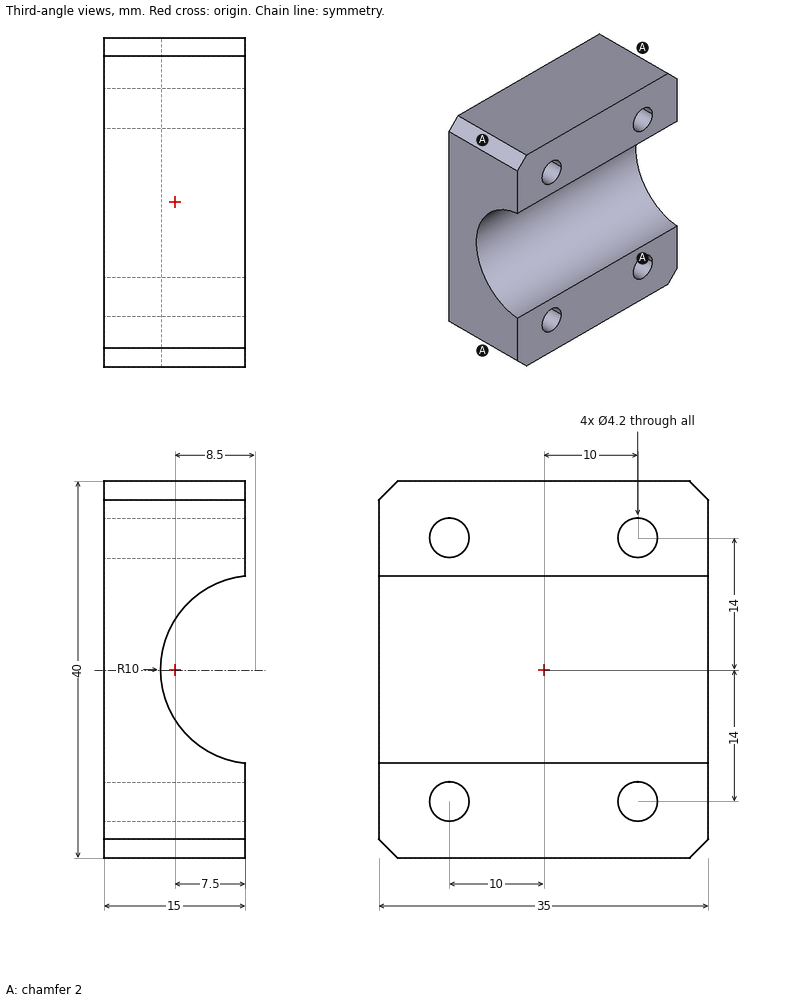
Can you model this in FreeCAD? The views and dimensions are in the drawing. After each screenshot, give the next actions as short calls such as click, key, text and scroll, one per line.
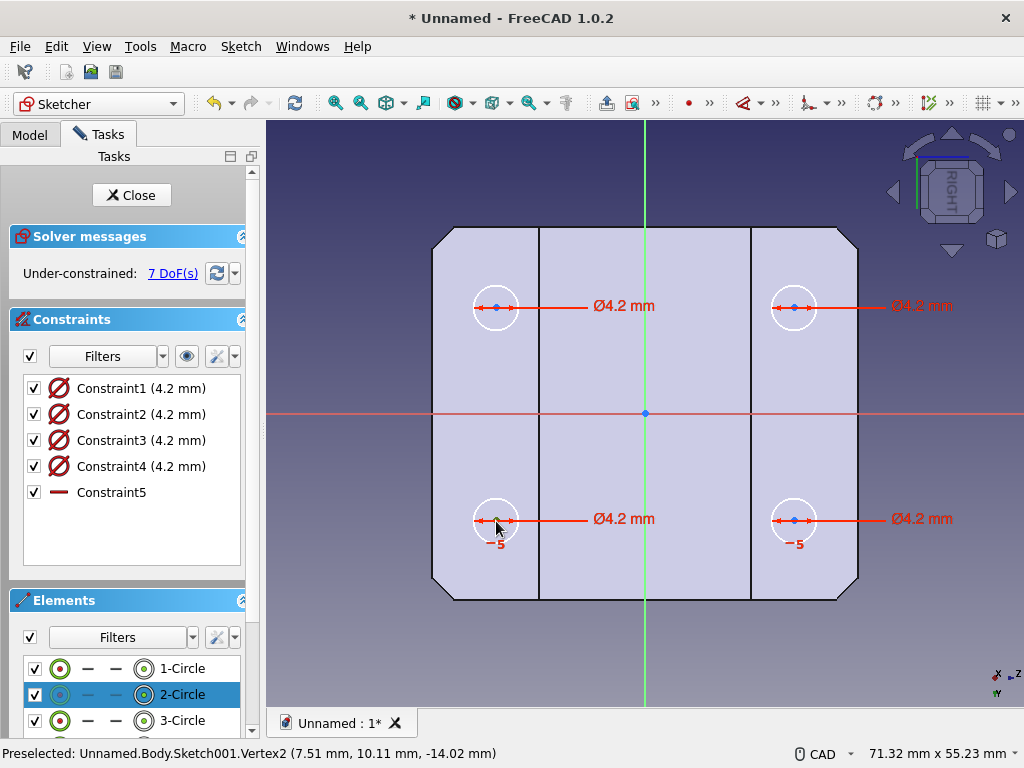
click(496, 308)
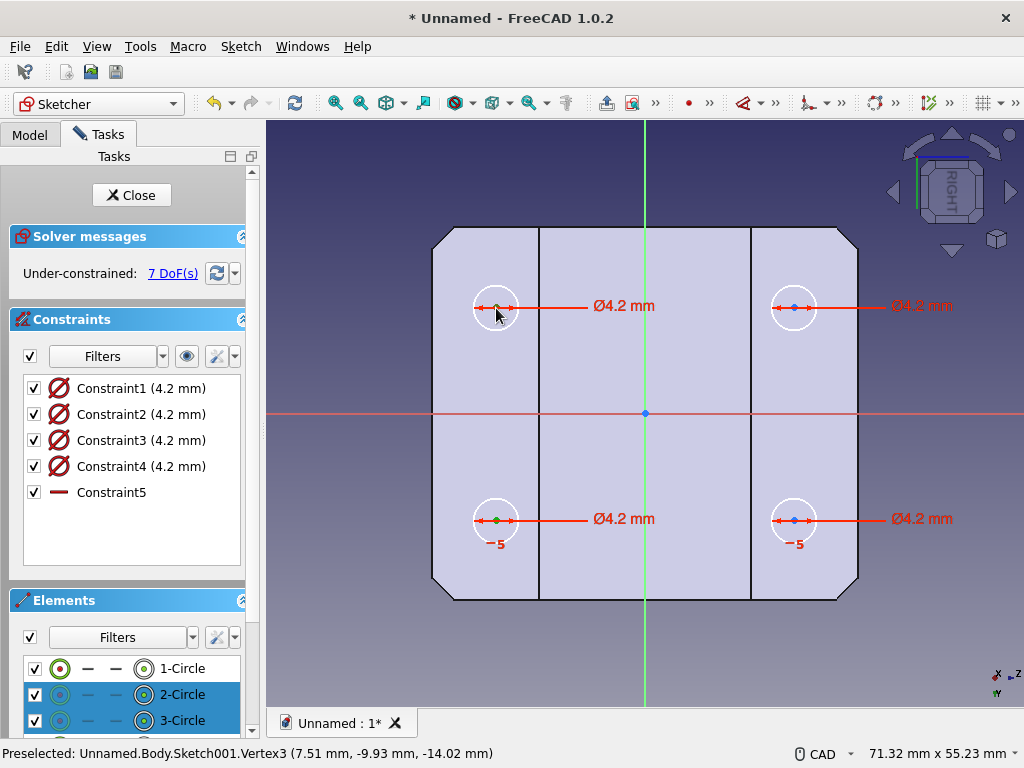
key(v)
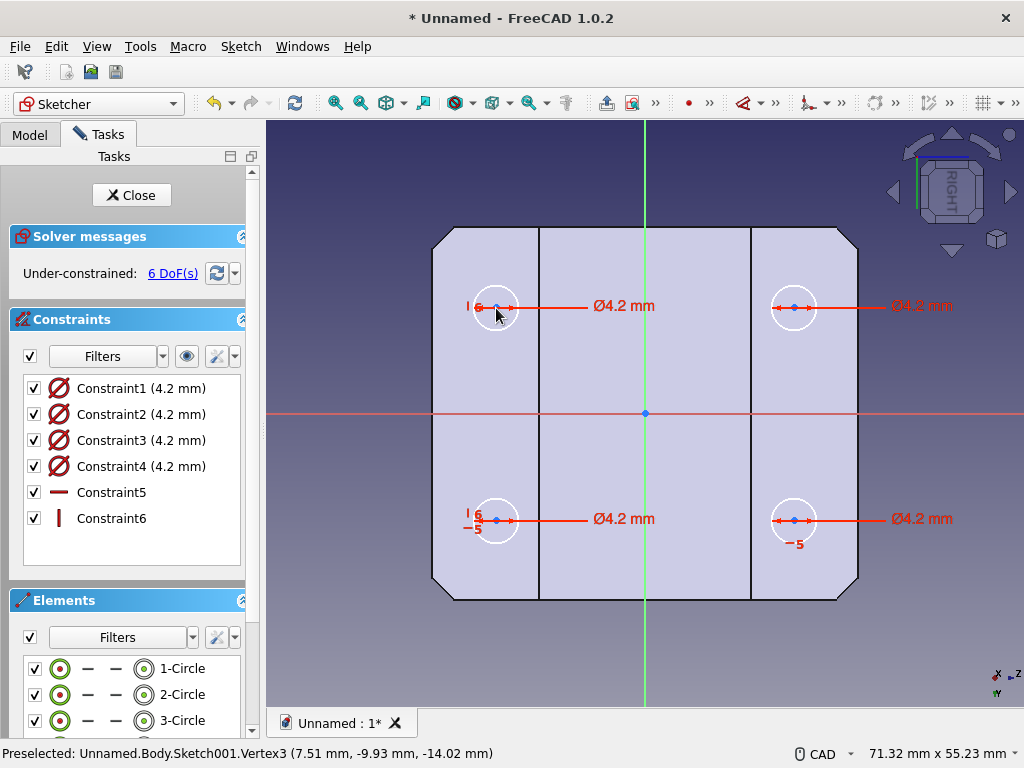
click(794, 521)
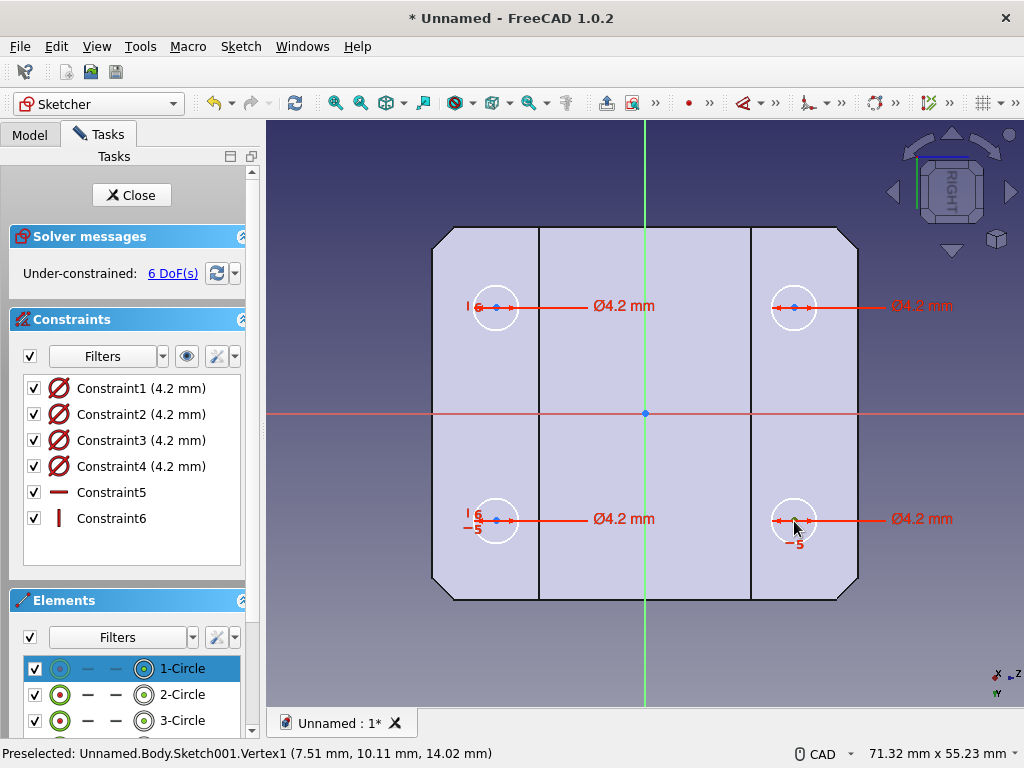
click(794, 308)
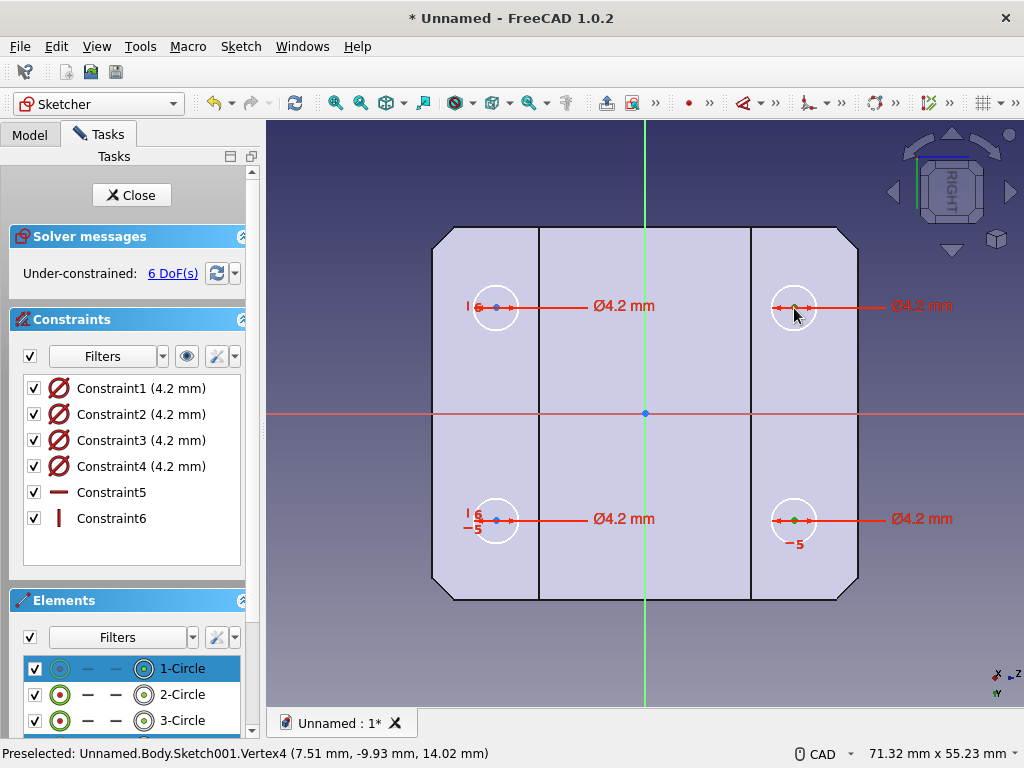
key(v)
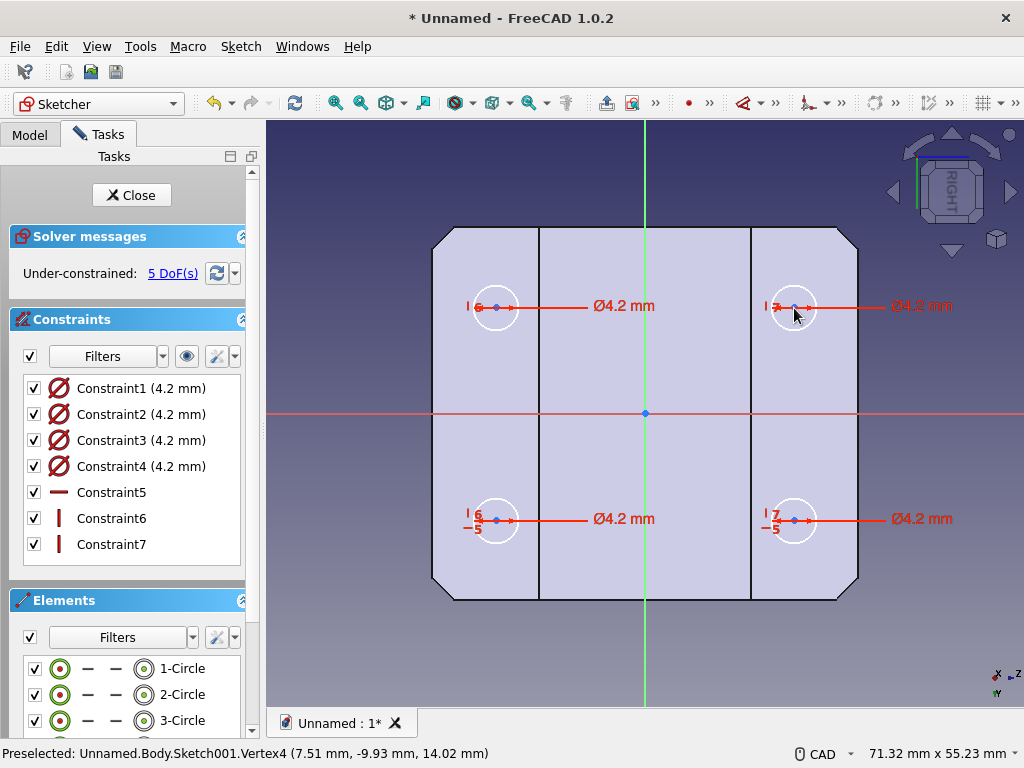
click(496, 308)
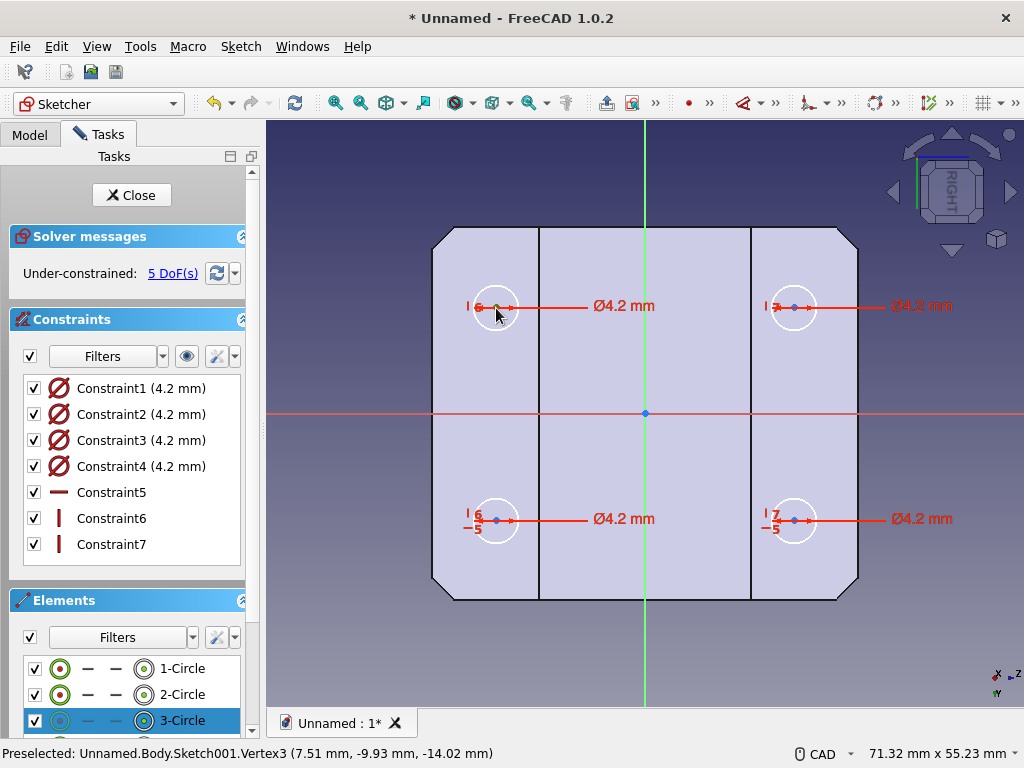
click(794, 308)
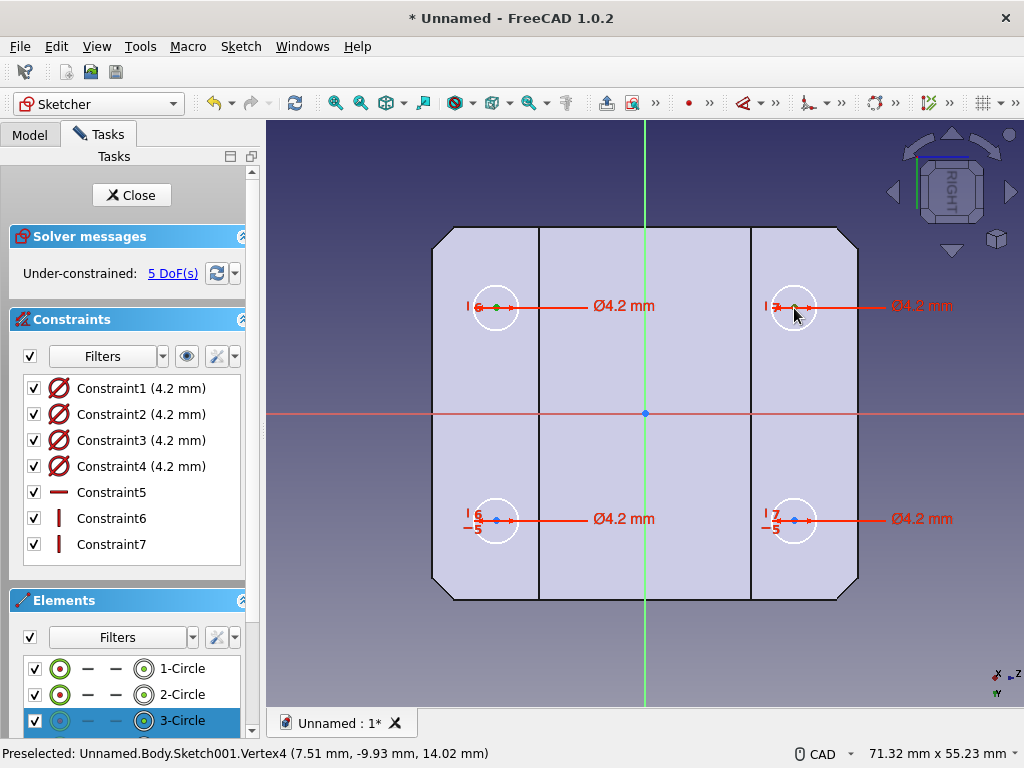
key(h)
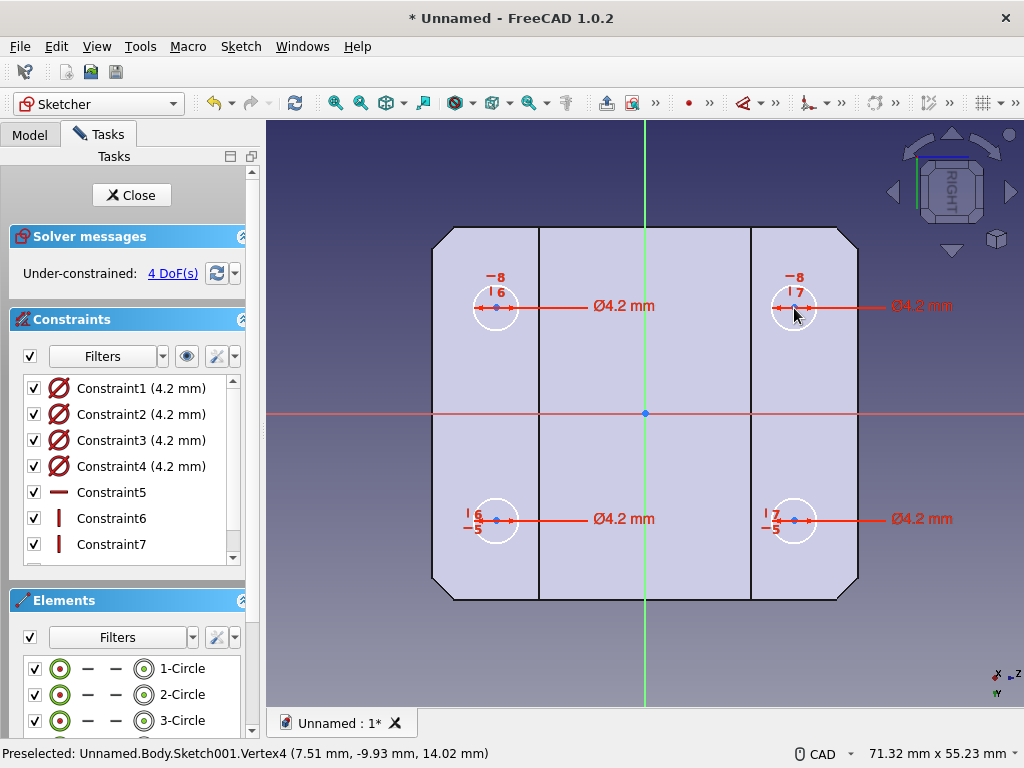
click(742, 104)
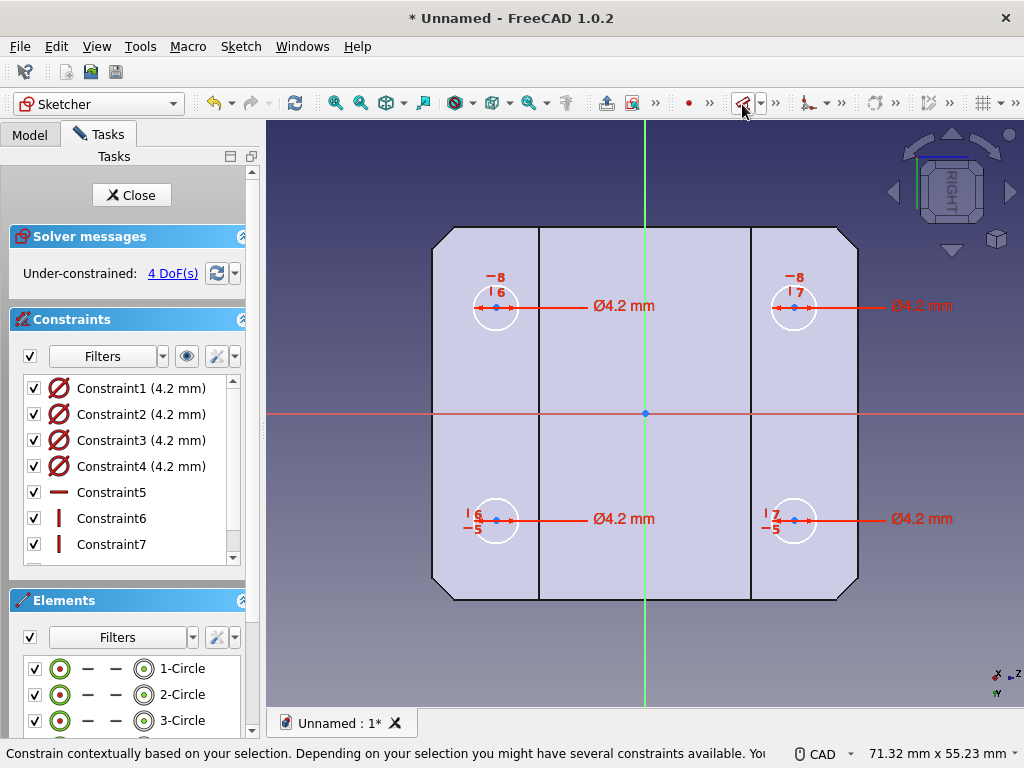
click(794, 521)
click(720, 555)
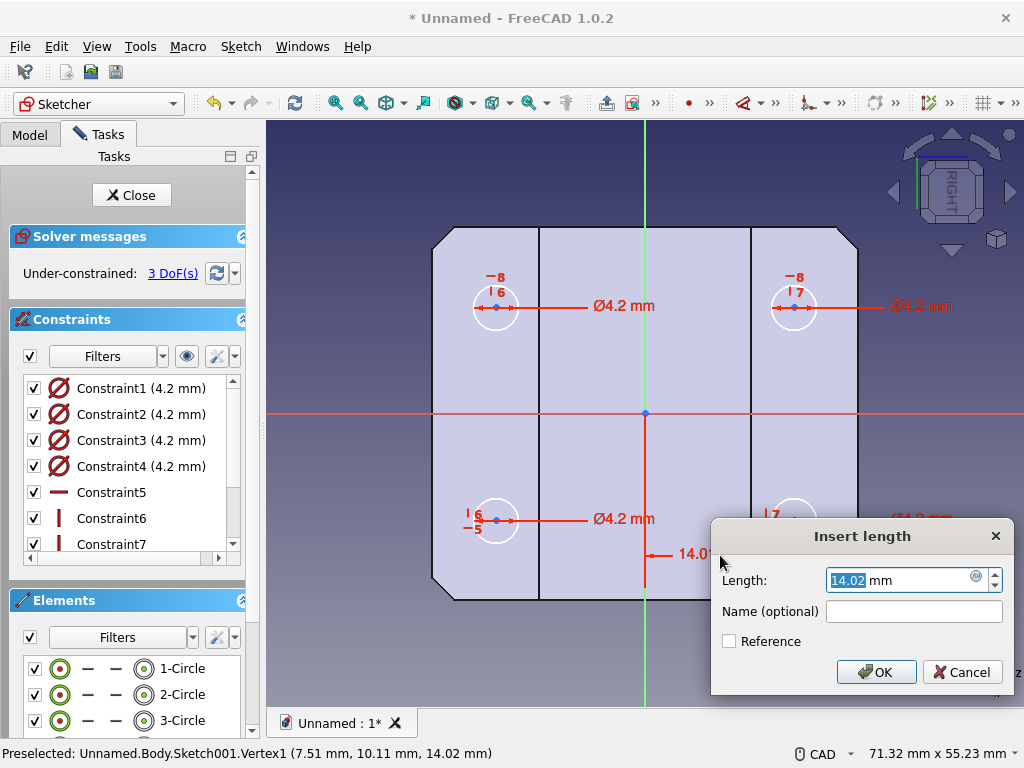
text(14)
key(Return)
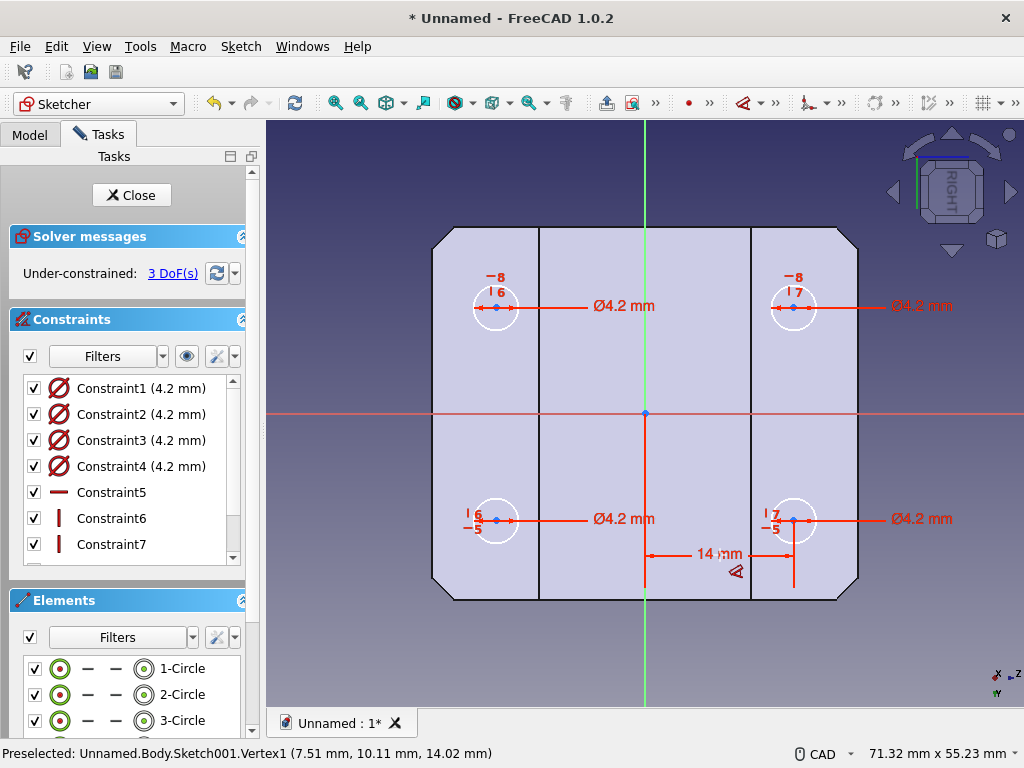
click(794, 521)
click(828, 467)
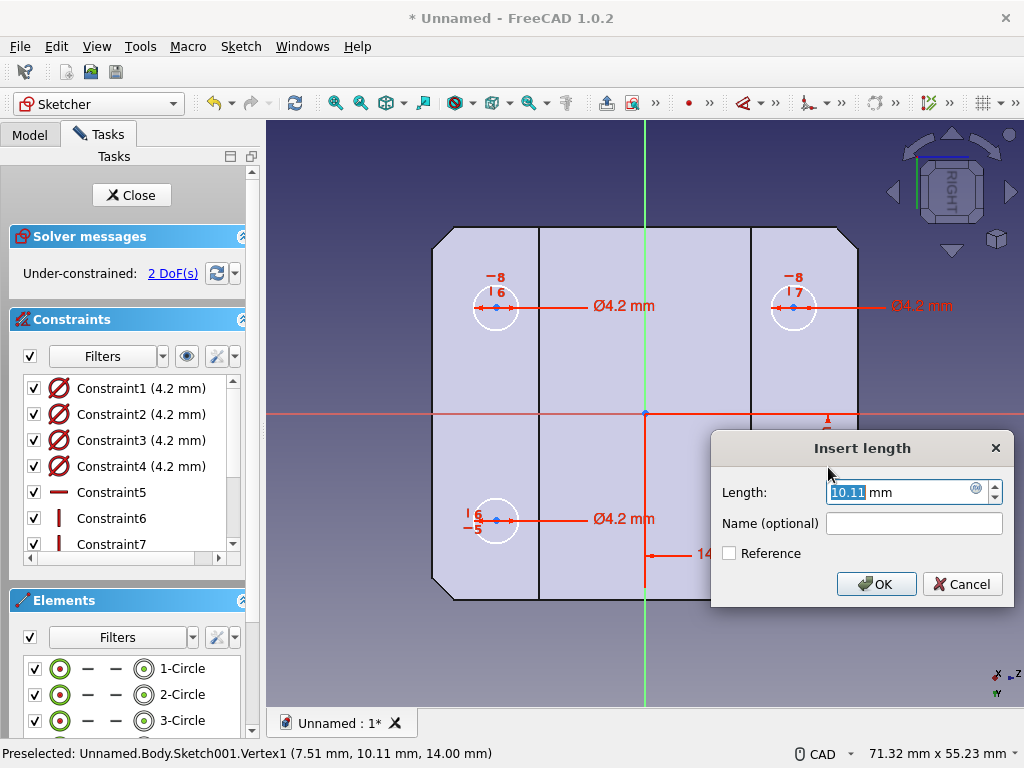
text(10)
key(Return)